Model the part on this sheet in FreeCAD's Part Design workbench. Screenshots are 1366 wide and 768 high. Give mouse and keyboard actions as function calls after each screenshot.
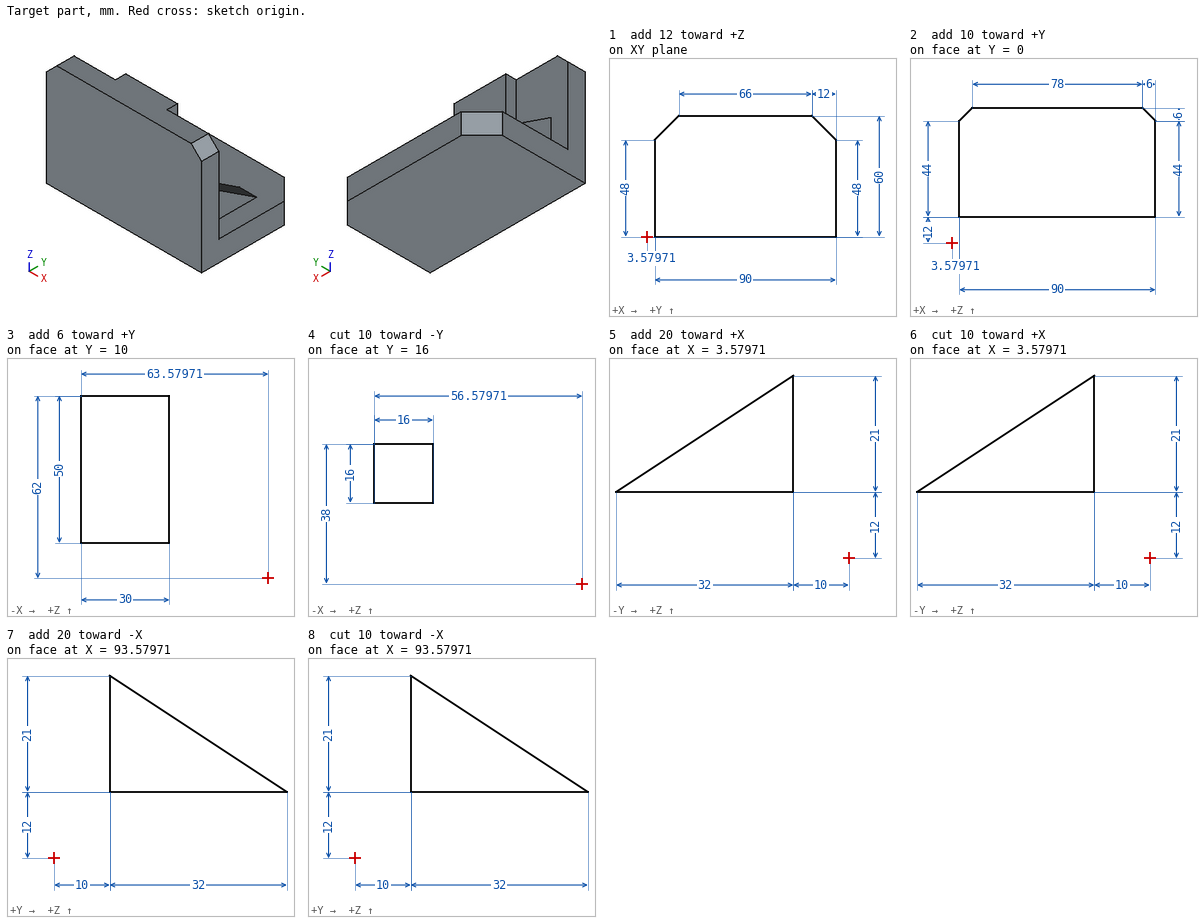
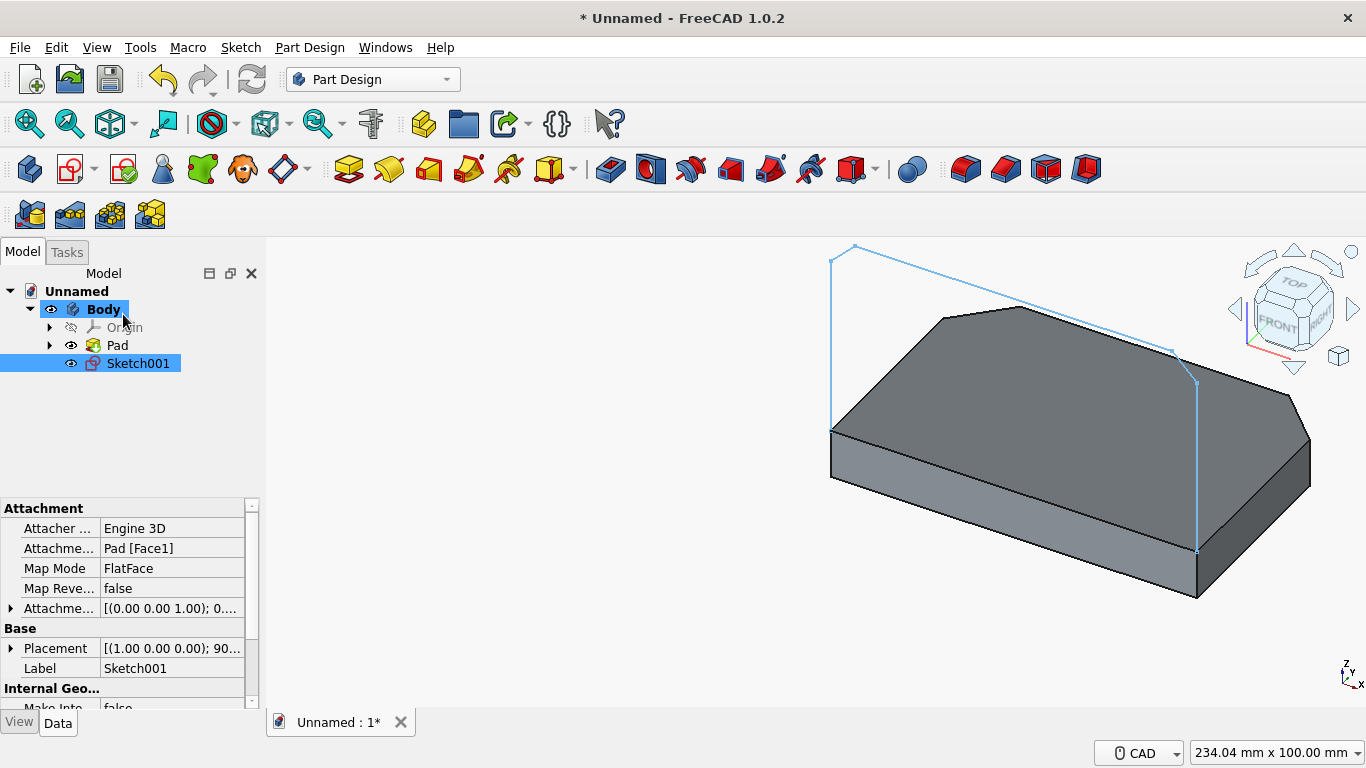
click(350, 170)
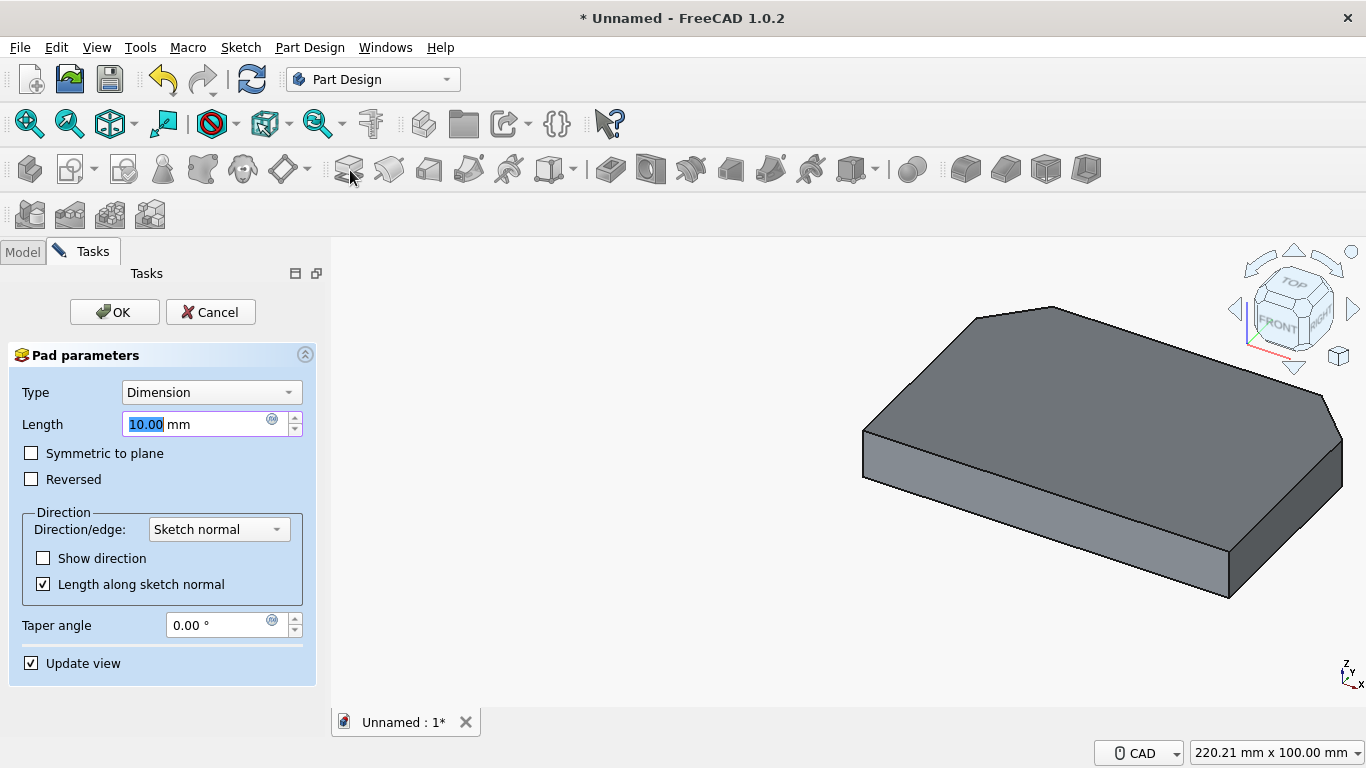
text(10)
key(Tab)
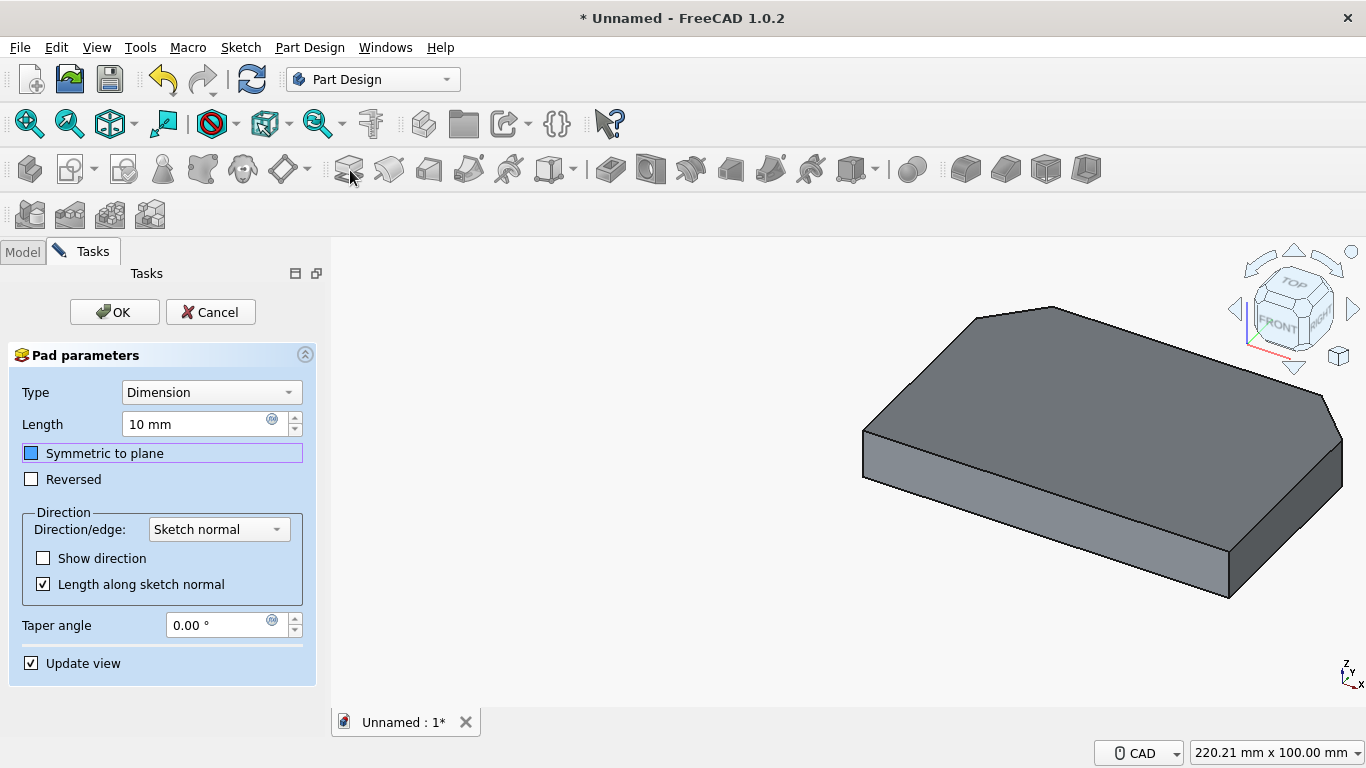
click(30, 479)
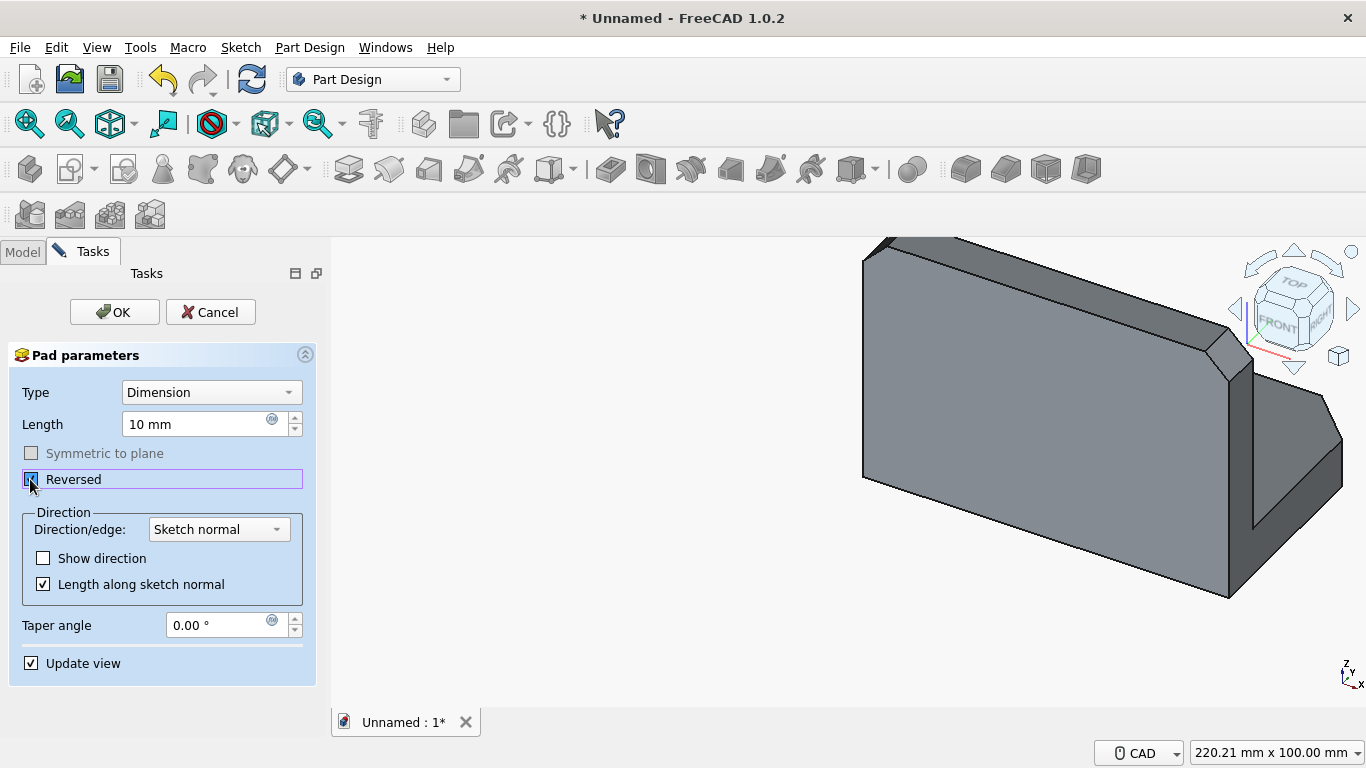
click(115, 312)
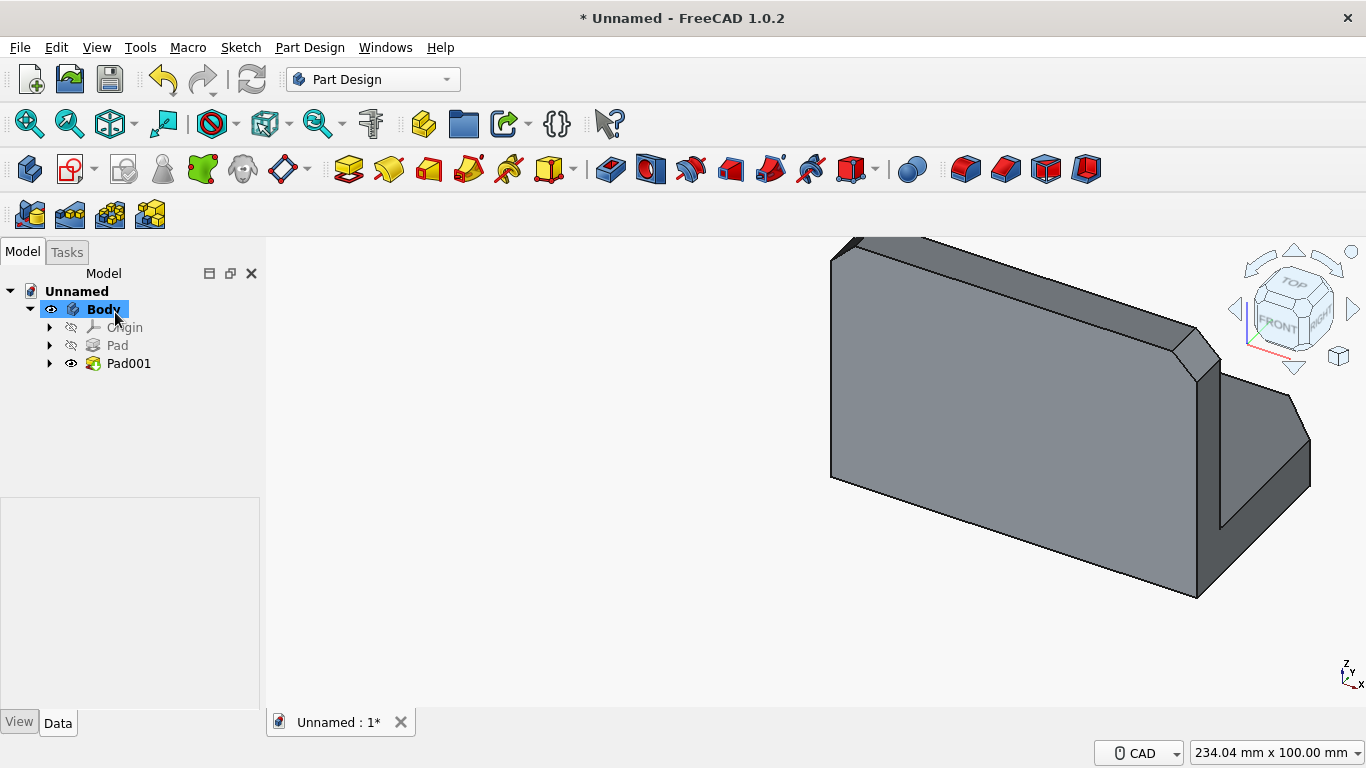
key(v)
key(f)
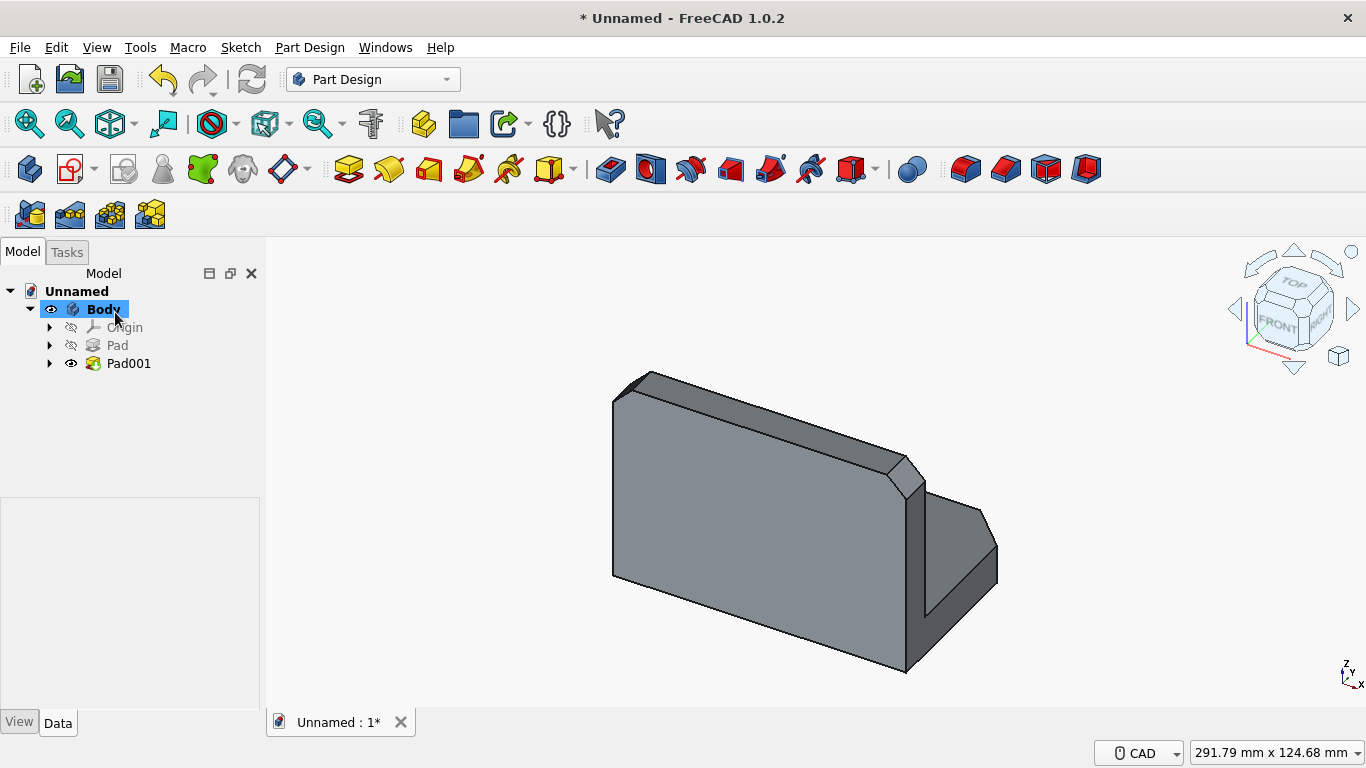
key(4)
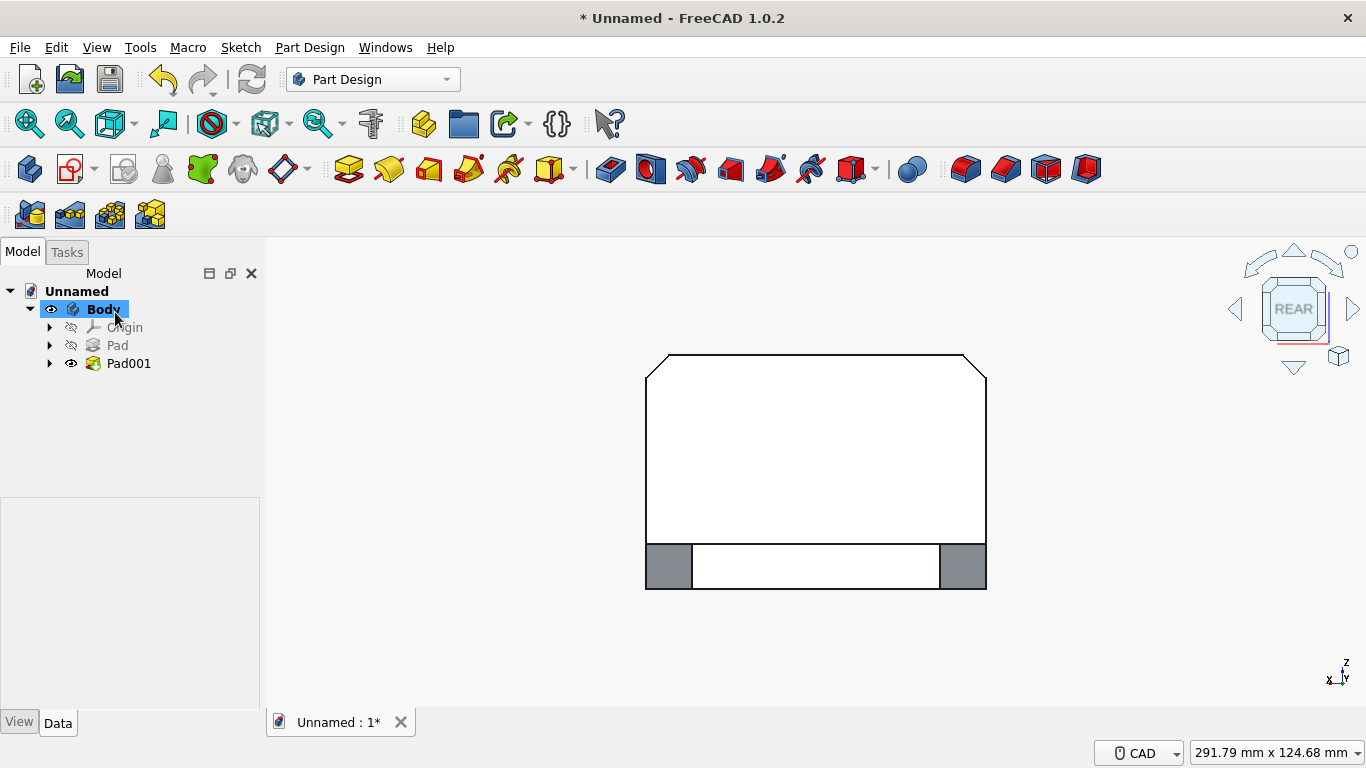
click(768, 448)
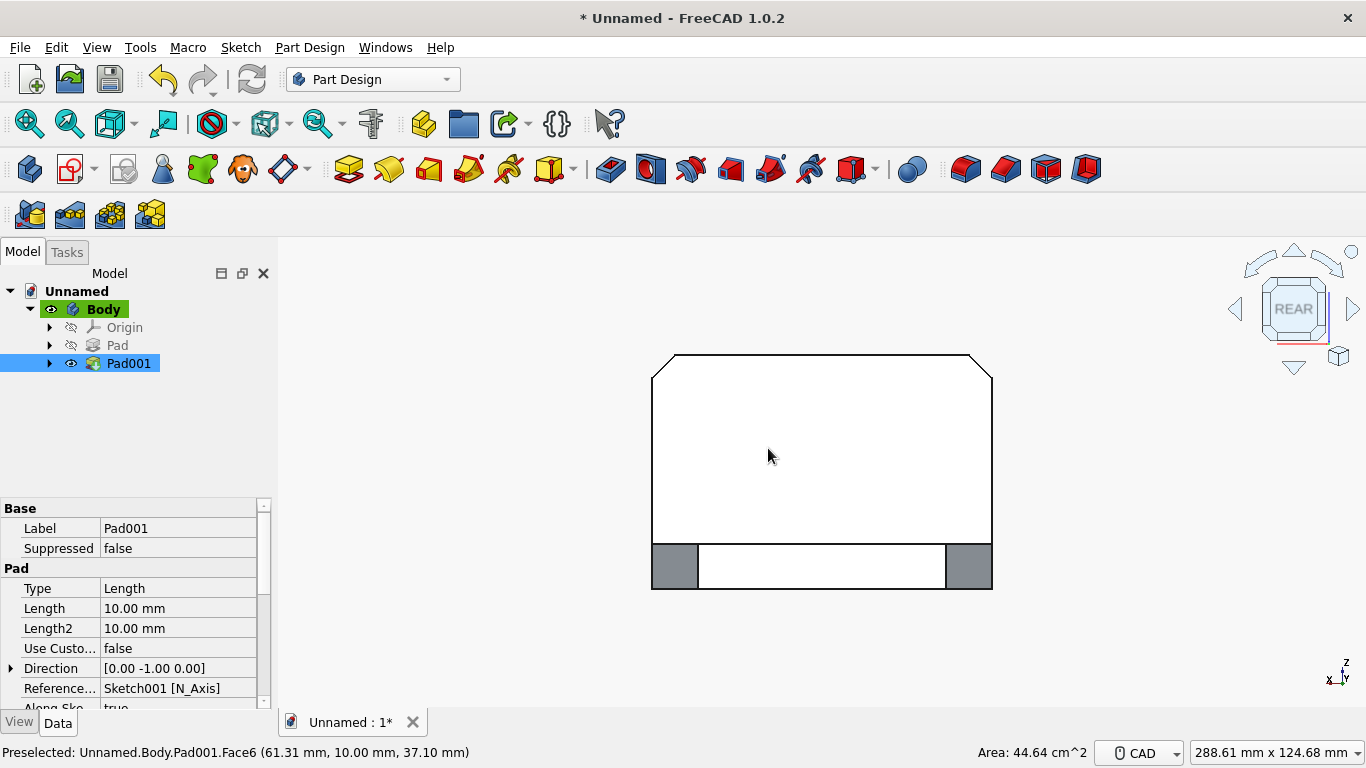
click(70, 170)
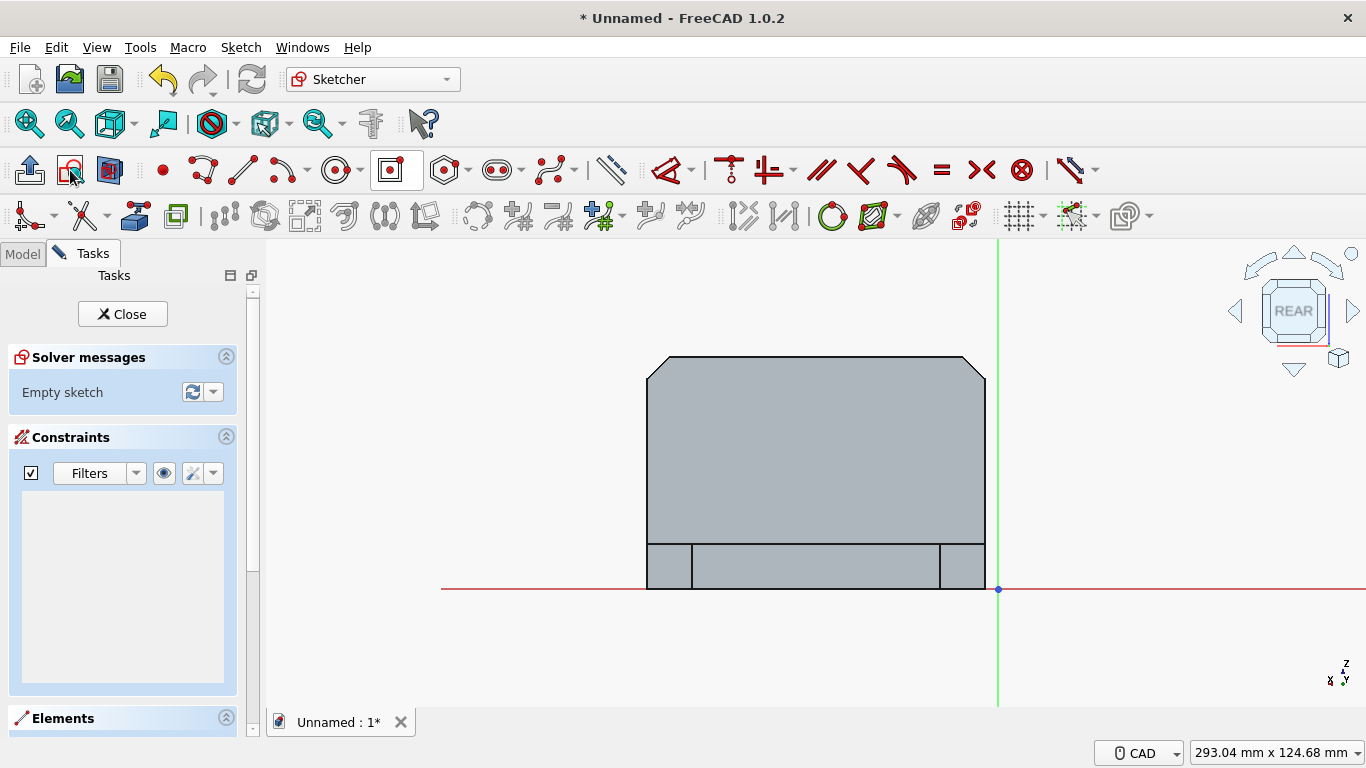
key(q)
key(s)